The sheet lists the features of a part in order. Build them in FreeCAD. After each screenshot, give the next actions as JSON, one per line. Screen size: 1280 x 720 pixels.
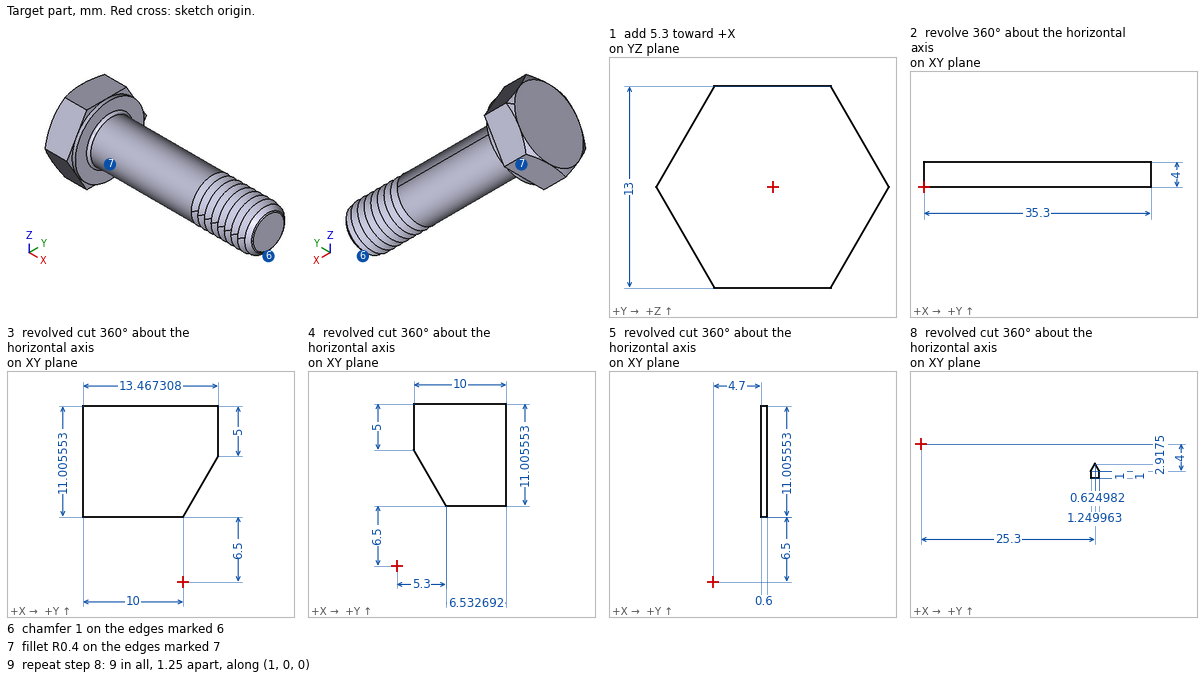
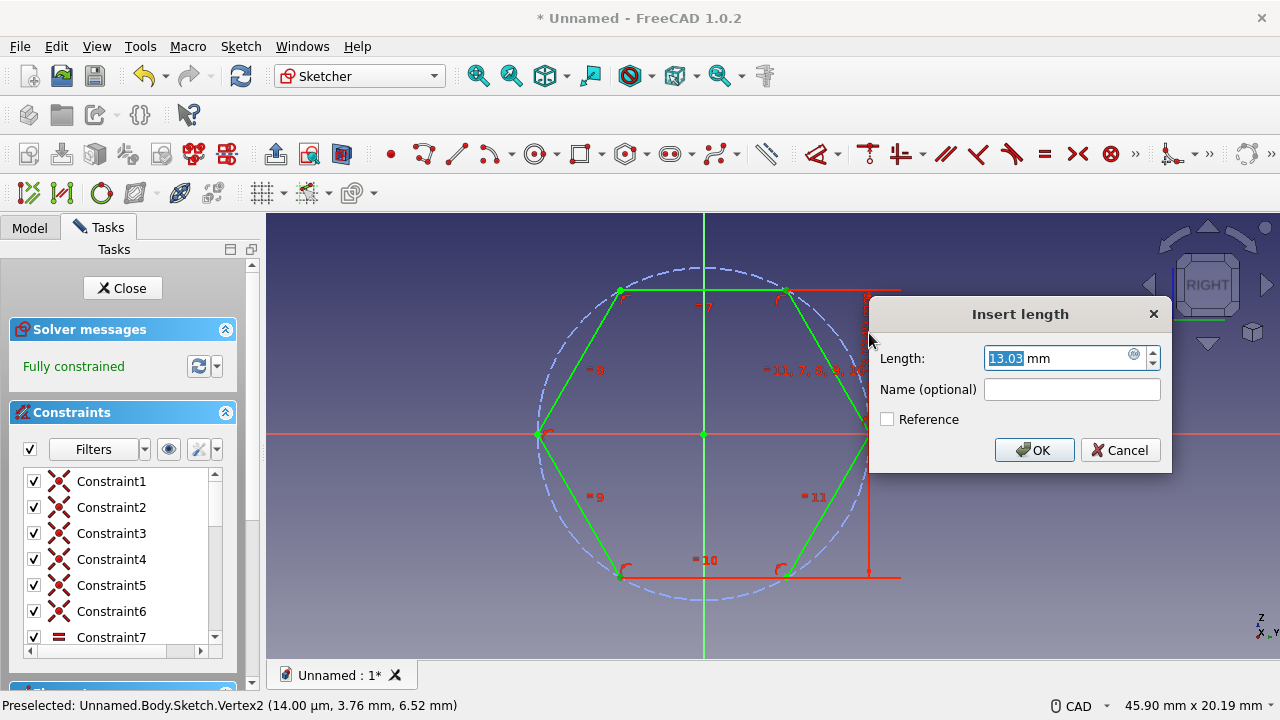
{"action": "type", "text": "13"}
{"action": "key", "text": "Return"}
{"action": "key", "text": "Escape"}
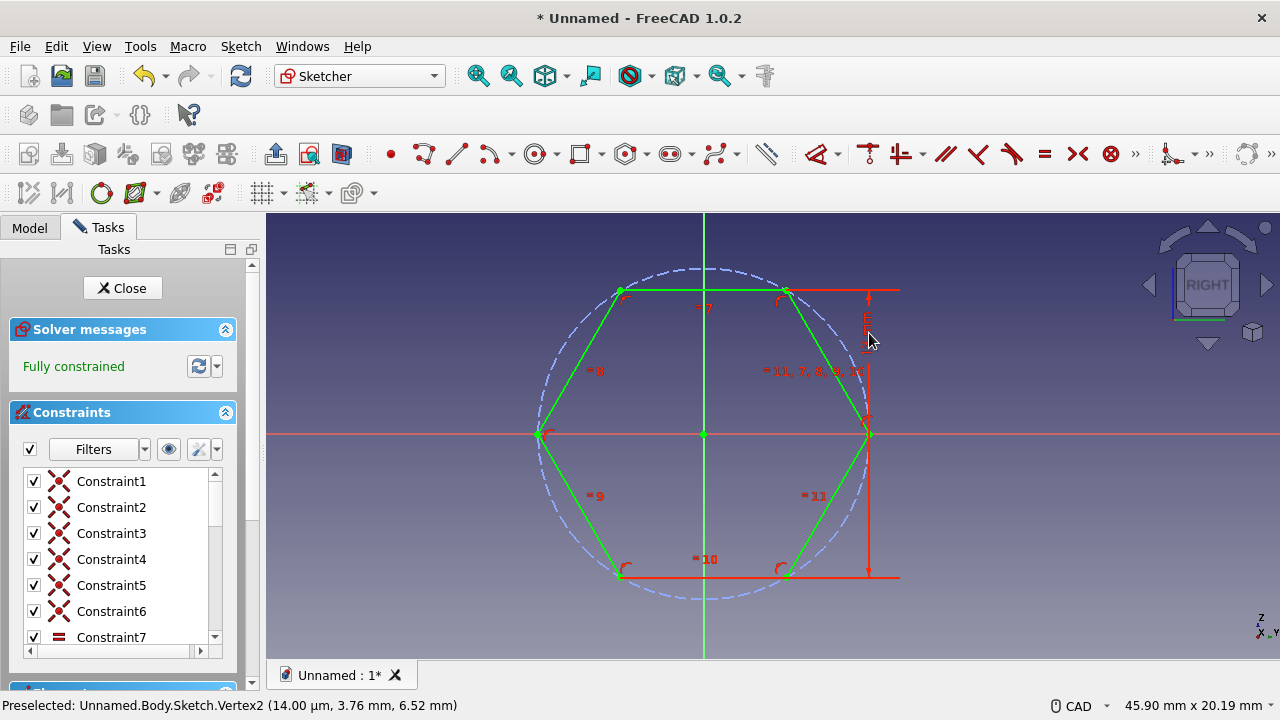
{"action": "left_click", "coordinate": [123, 288]}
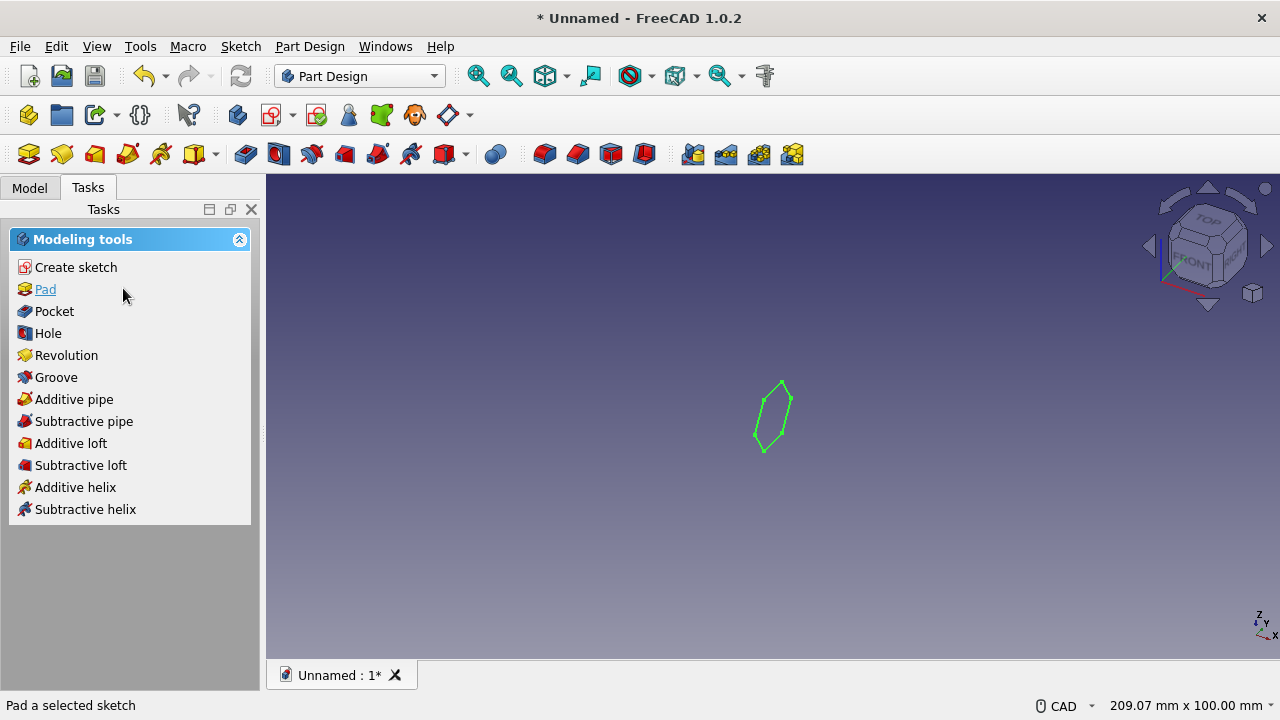
{"action": "left_click", "coordinate": [29, 154]}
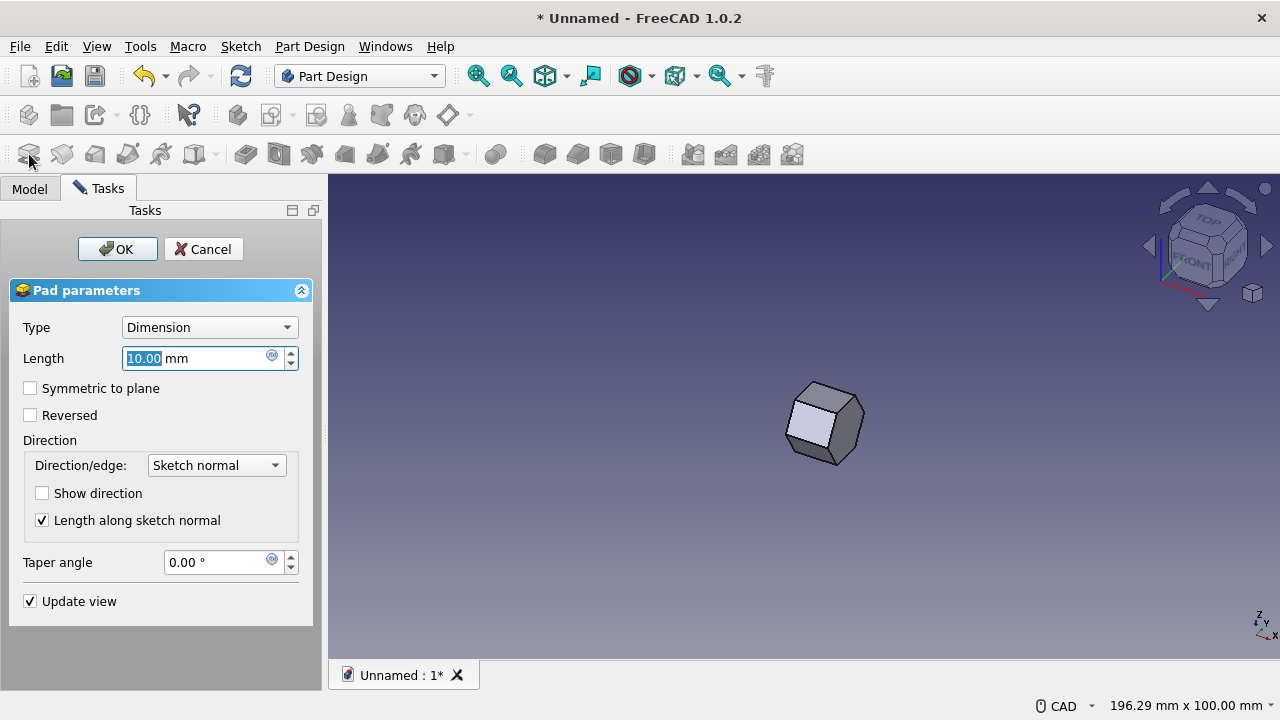
{"action": "type", "text": "5.3"}
{"action": "key", "text": "Tab"}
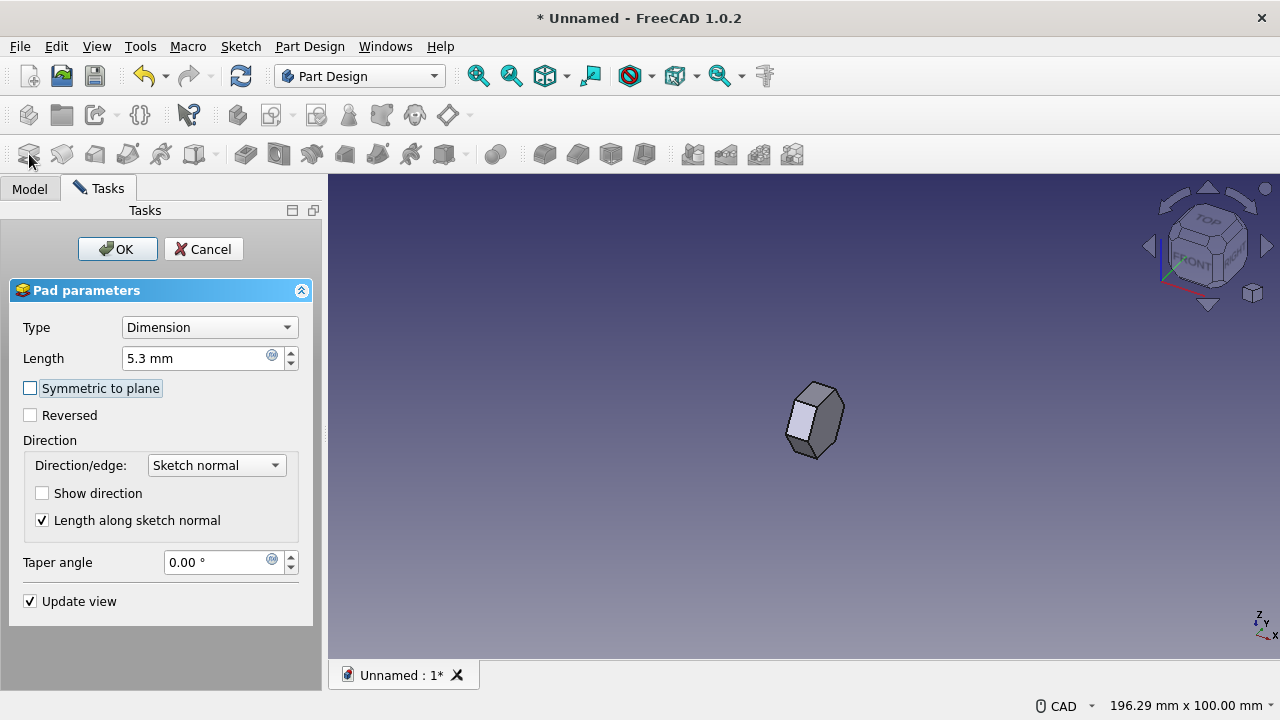
{"action": "left_click", "coordinate": [118, 249]}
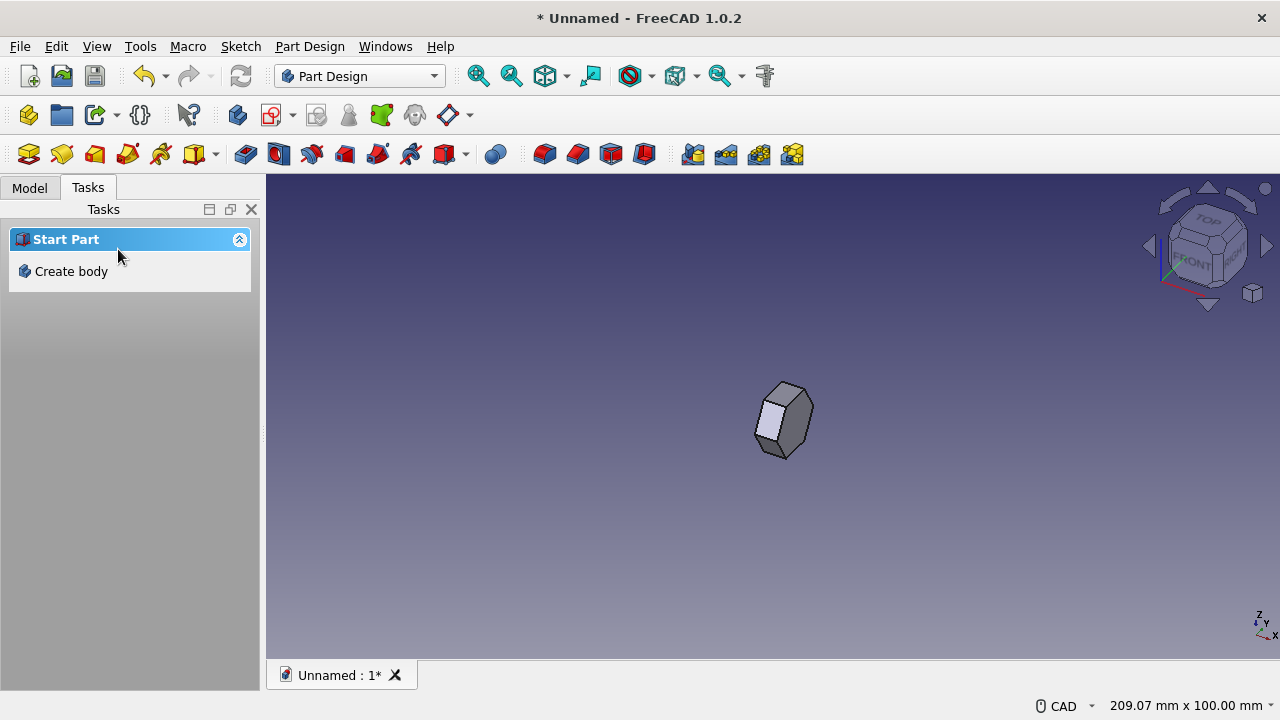
{"action": "left_click", "coordinate": [479, 76]}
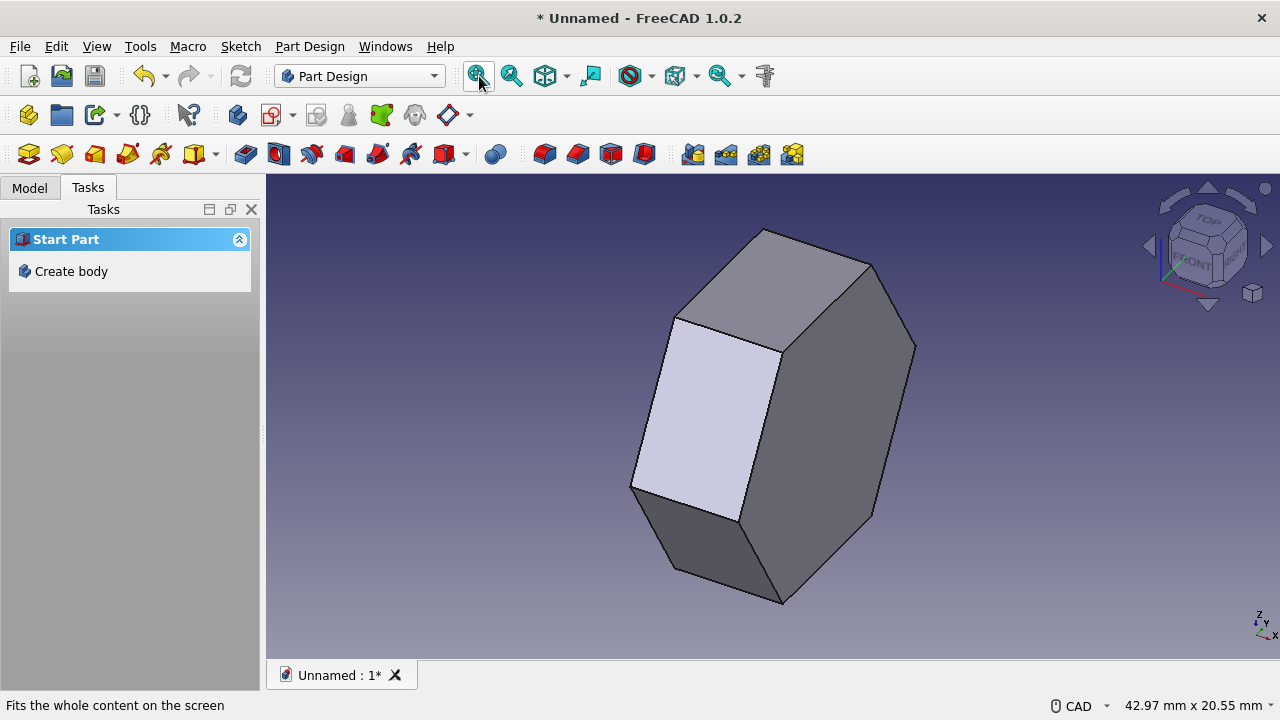
{"action": "left_click", "coordinate": [270, 116]}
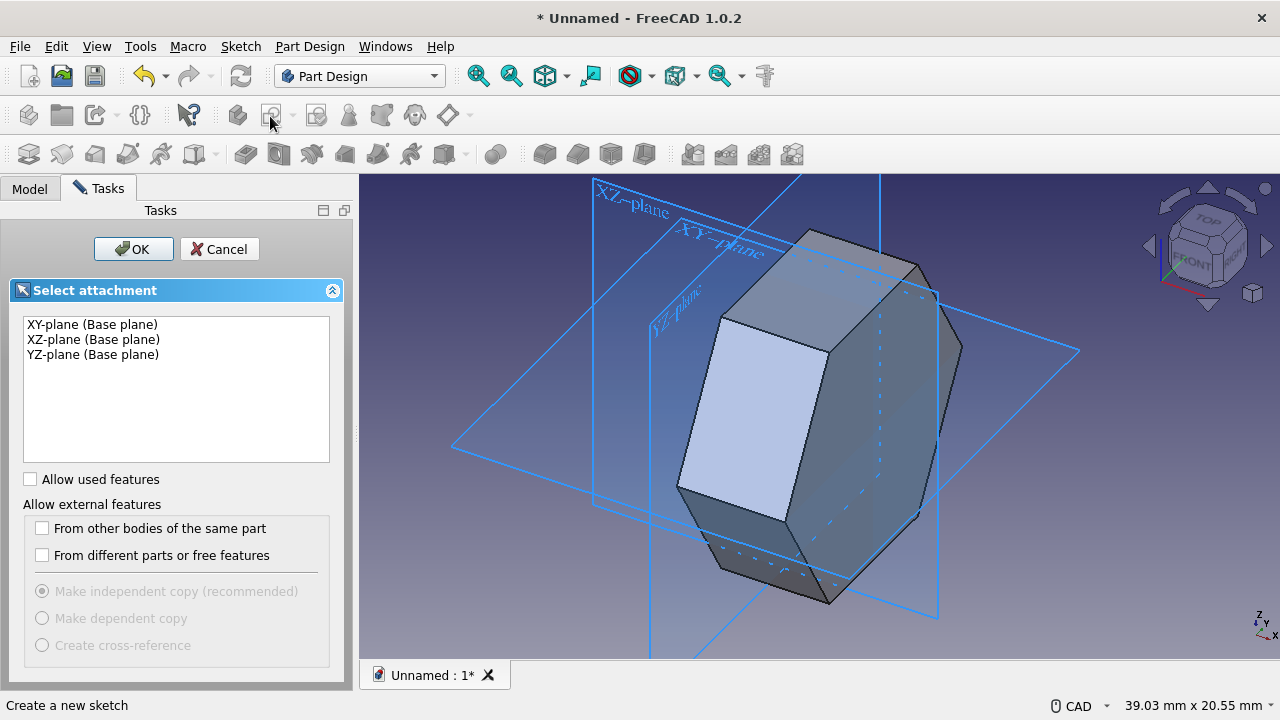
{"action": "left_click", "coordinate": [84, 324]}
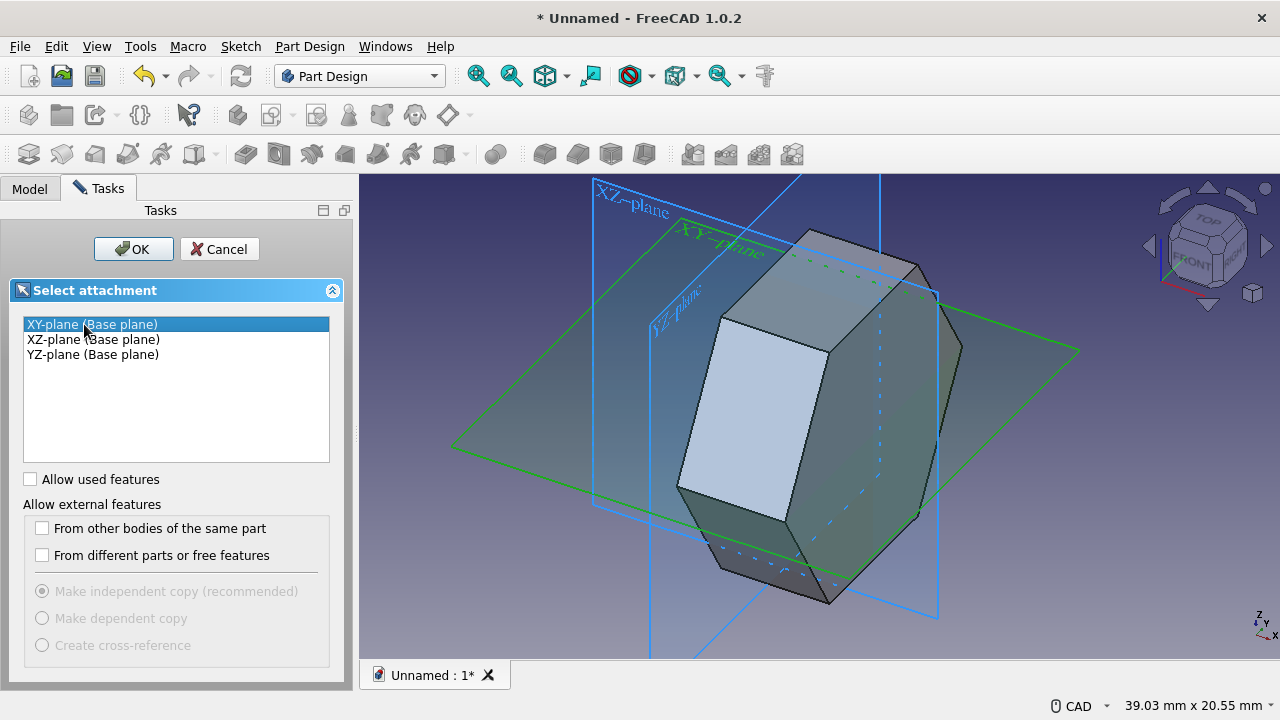
{"action": "left_click", "coordinate": [134, 249]}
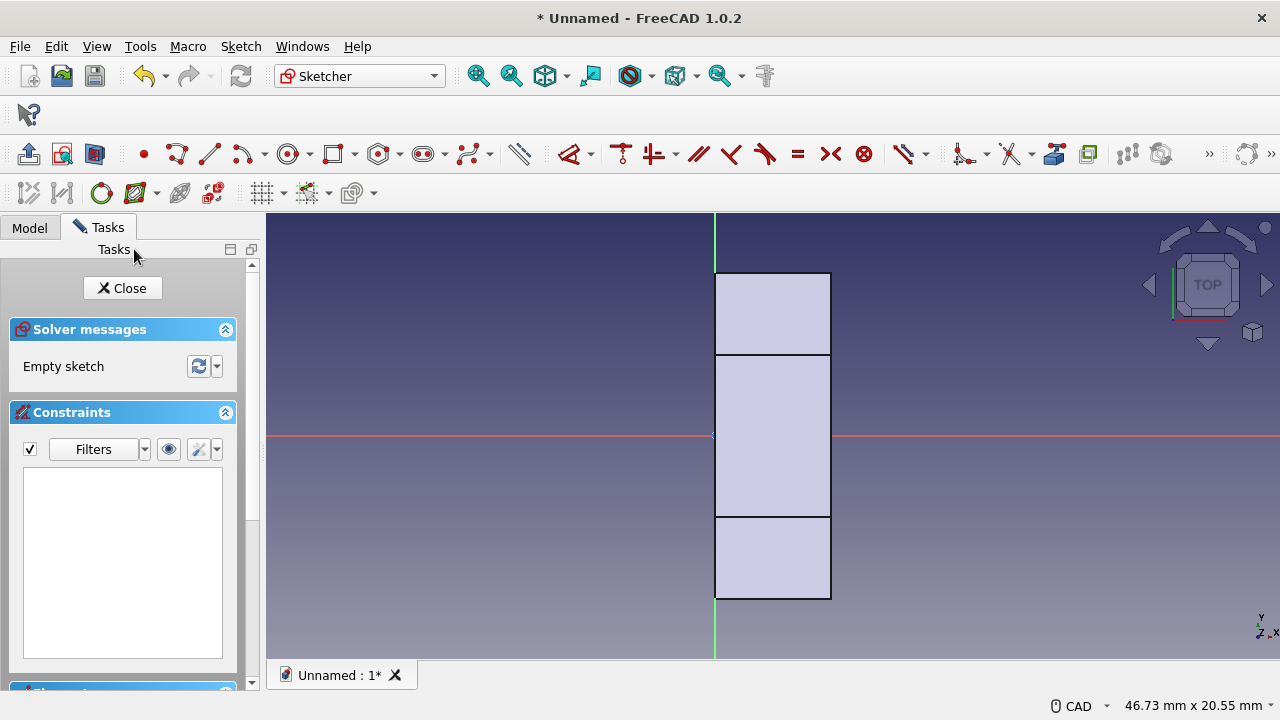
{"action": "left_click", "coordinate": [95, 154]}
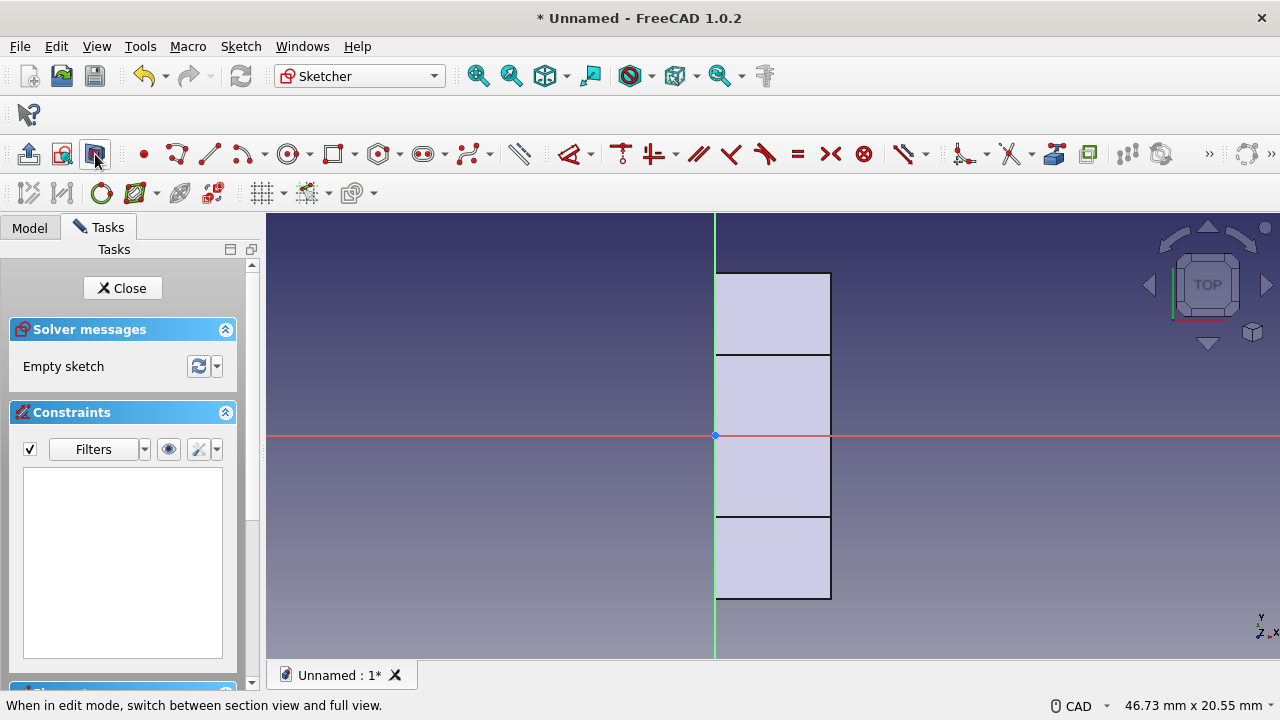
{"action": "scroll", "coordinate": [294, 489], "scroll_direction": "down", "scroll_amount": 3}